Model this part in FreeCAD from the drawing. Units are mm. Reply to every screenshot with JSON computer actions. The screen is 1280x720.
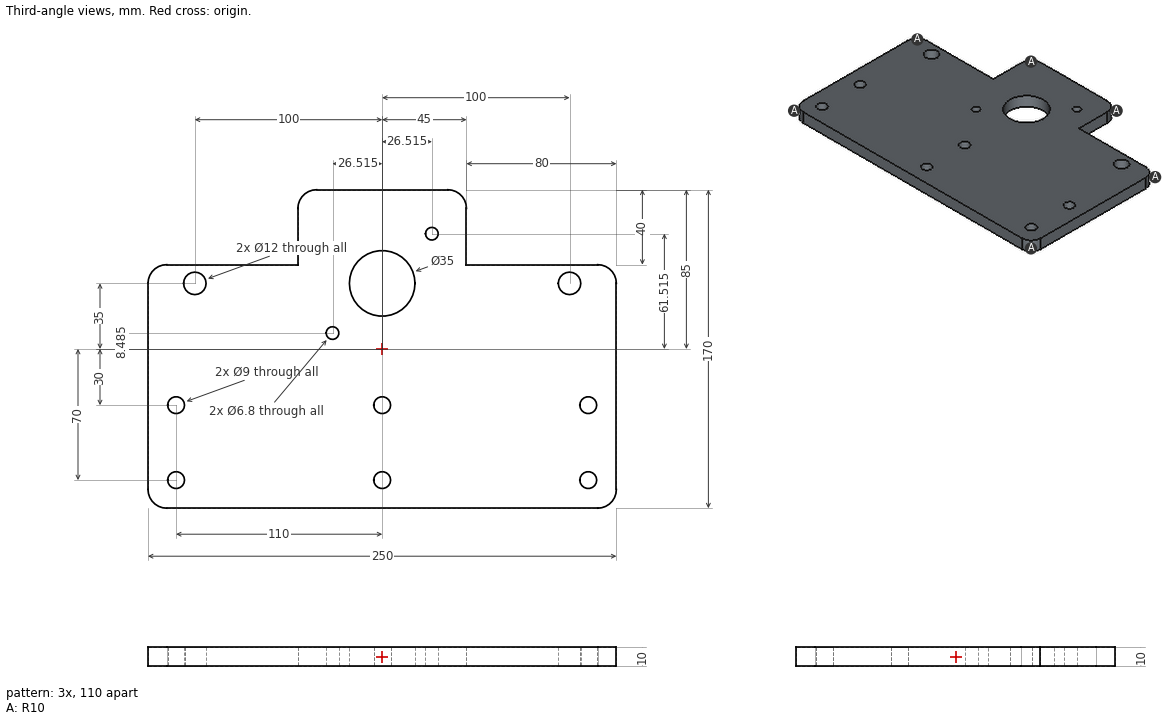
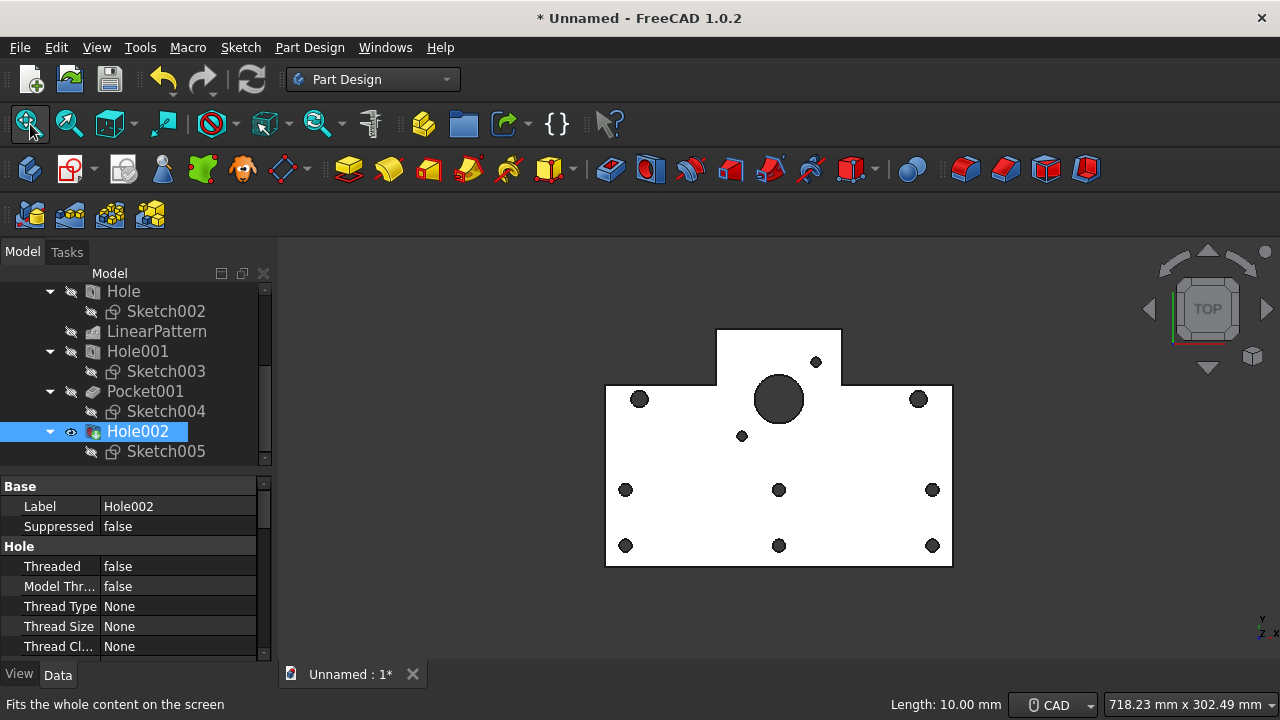
{"action": "key", "text": "1"}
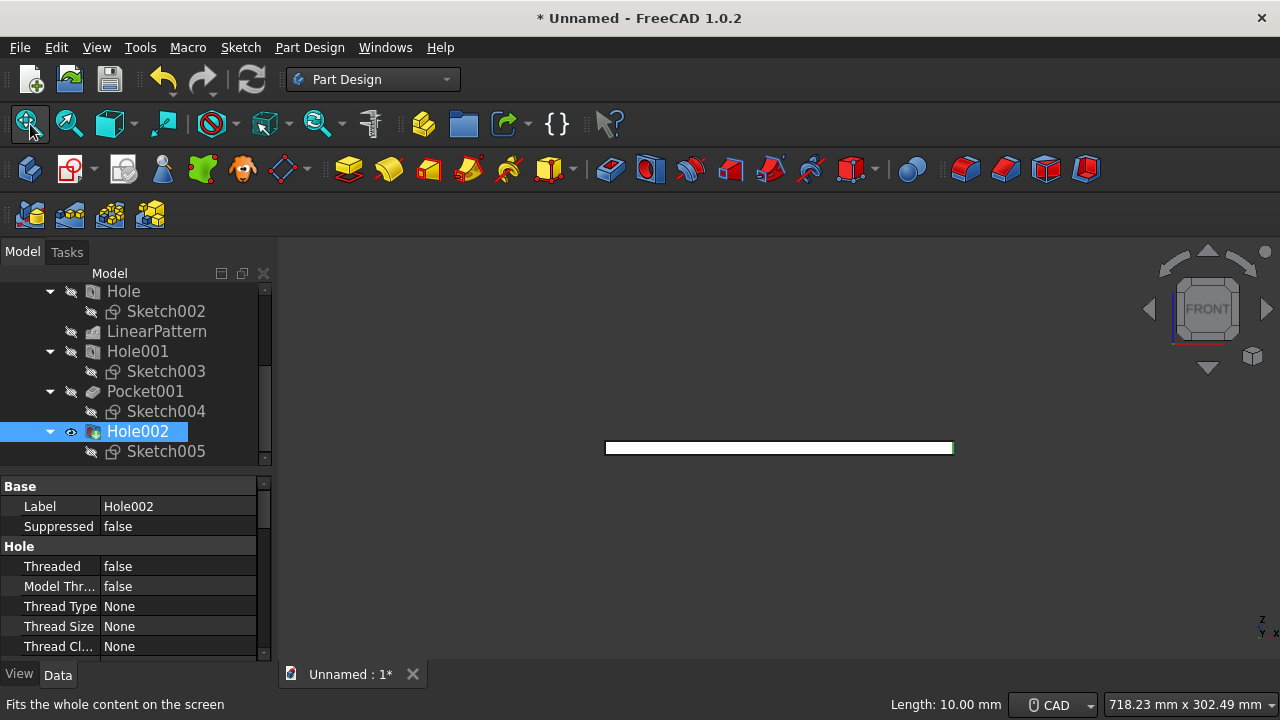
{"action": "left_click", "coordinate": [30, 124]}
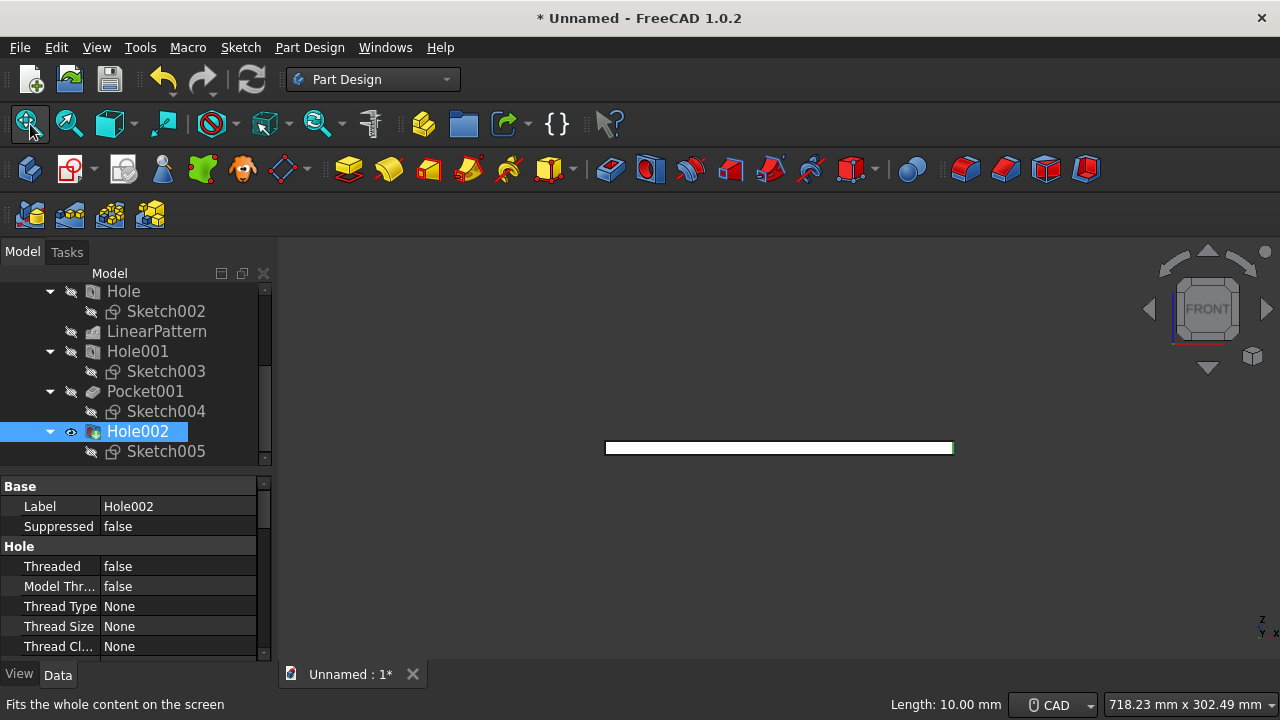
{"action": "left_click", "coordinate": [605, 447], "text": "ctrl"}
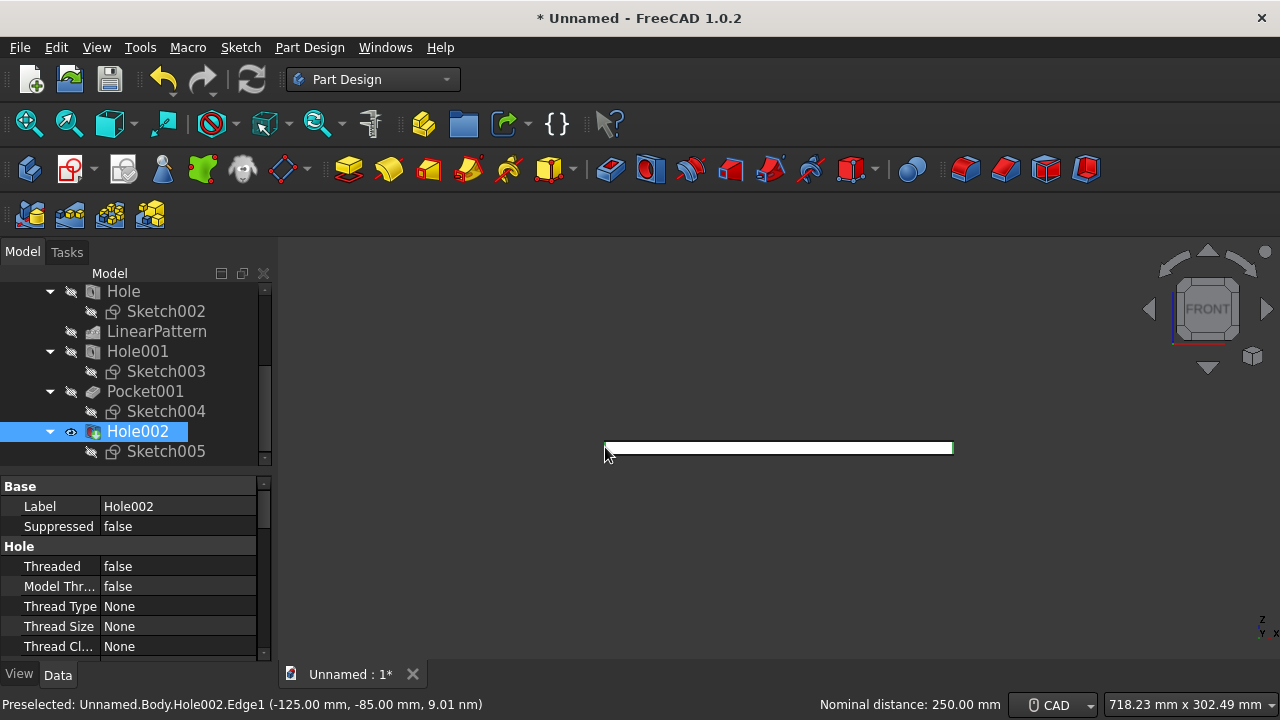
{"action": "scroll", "coordinate": [842, 447], "scroll_direction": "up", "scroll_amount": 6}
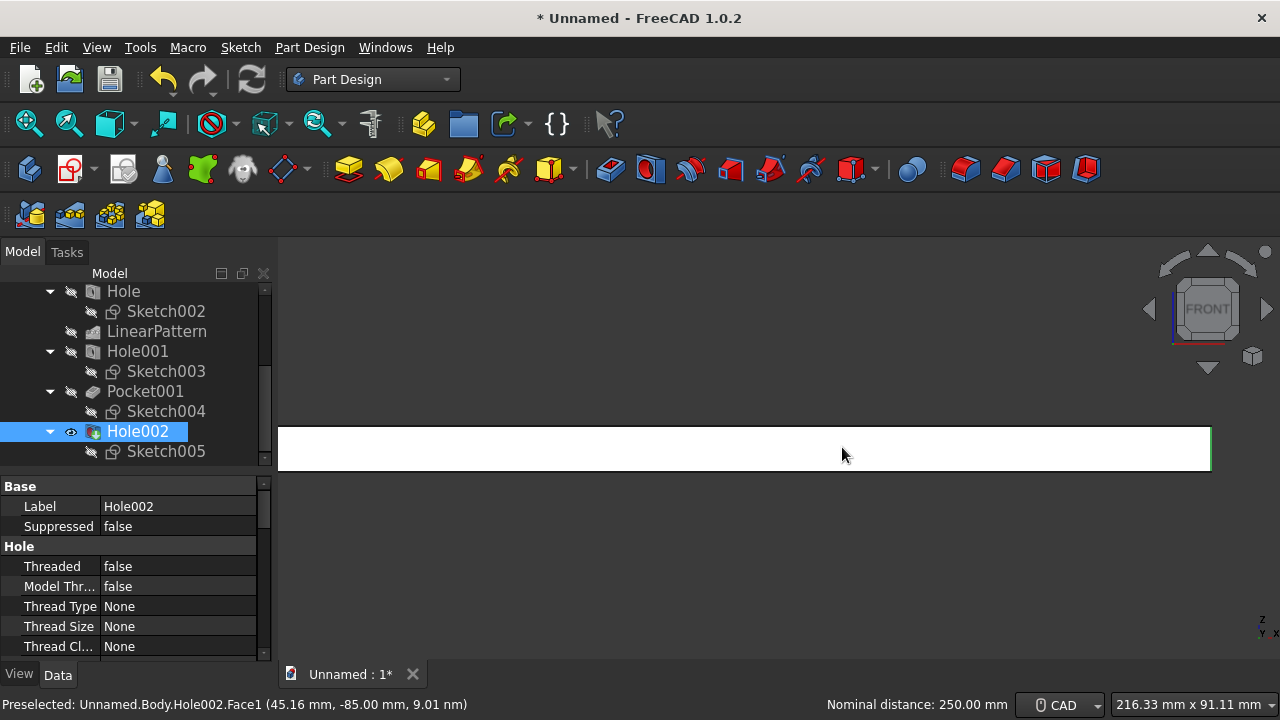
{"action": "left_click", "coordinate": [30, 124]}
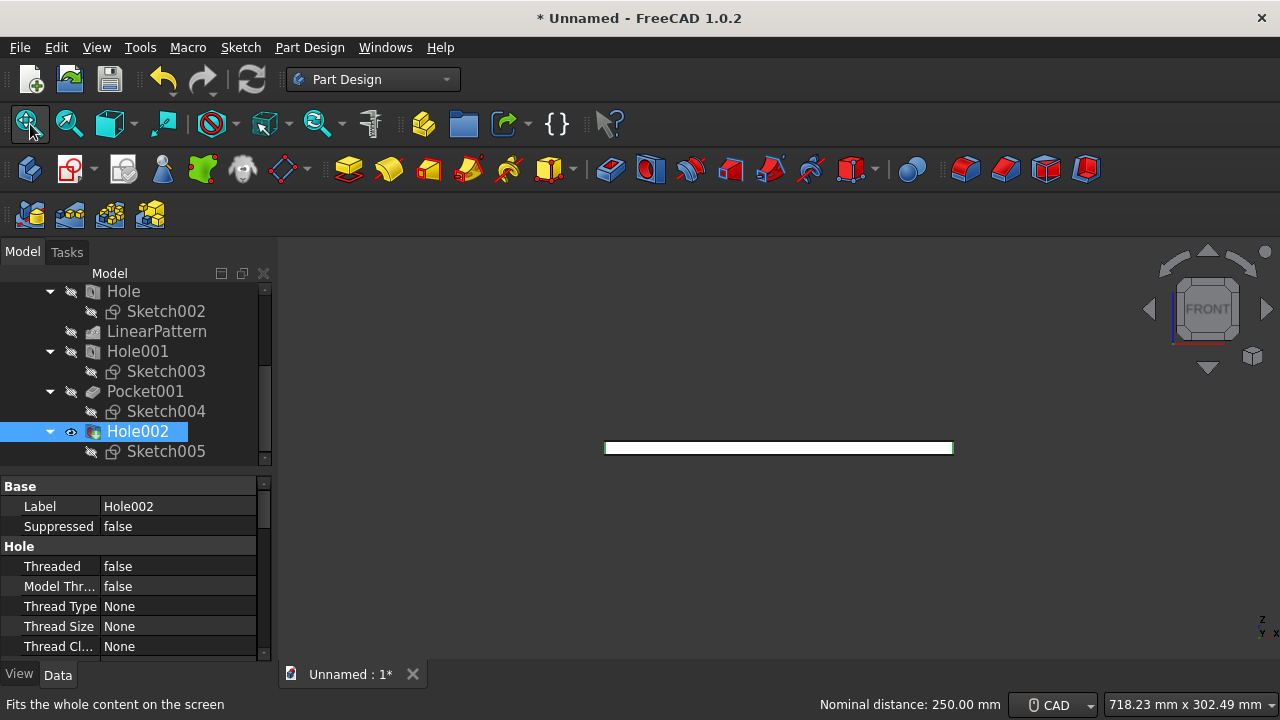
{"action": "key", "text": "3"}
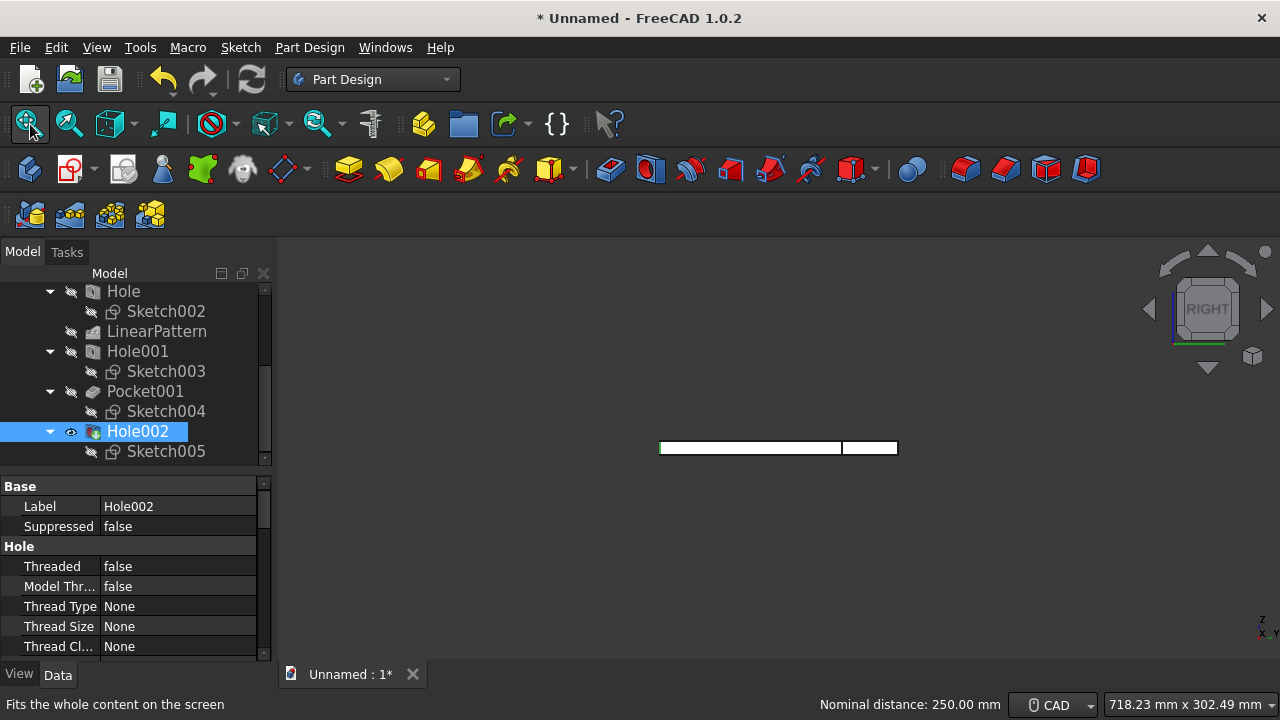
{"action": "left_click", "coordinate": [30, 124]}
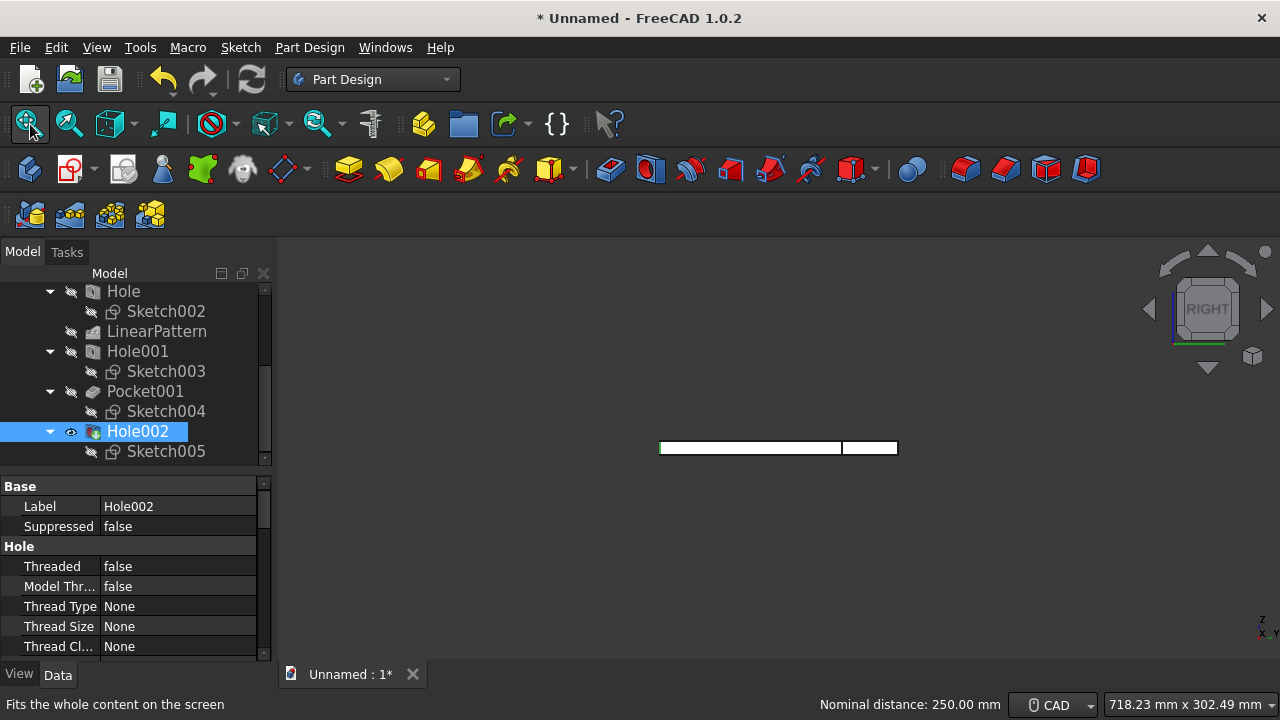
{"action": "left_click", "coordinate": [898, 447], "text": "ctrl"}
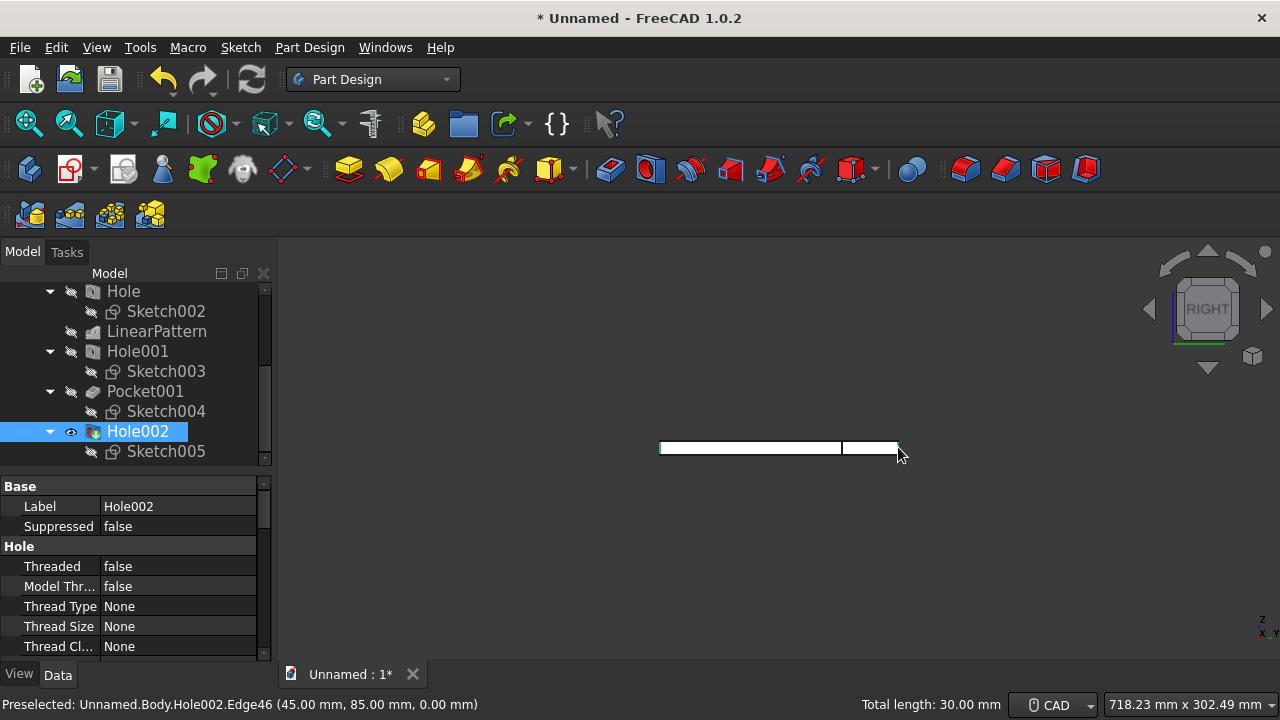
{"action": "left_click", "coordinate": [842, 447], "text": "ctrl"}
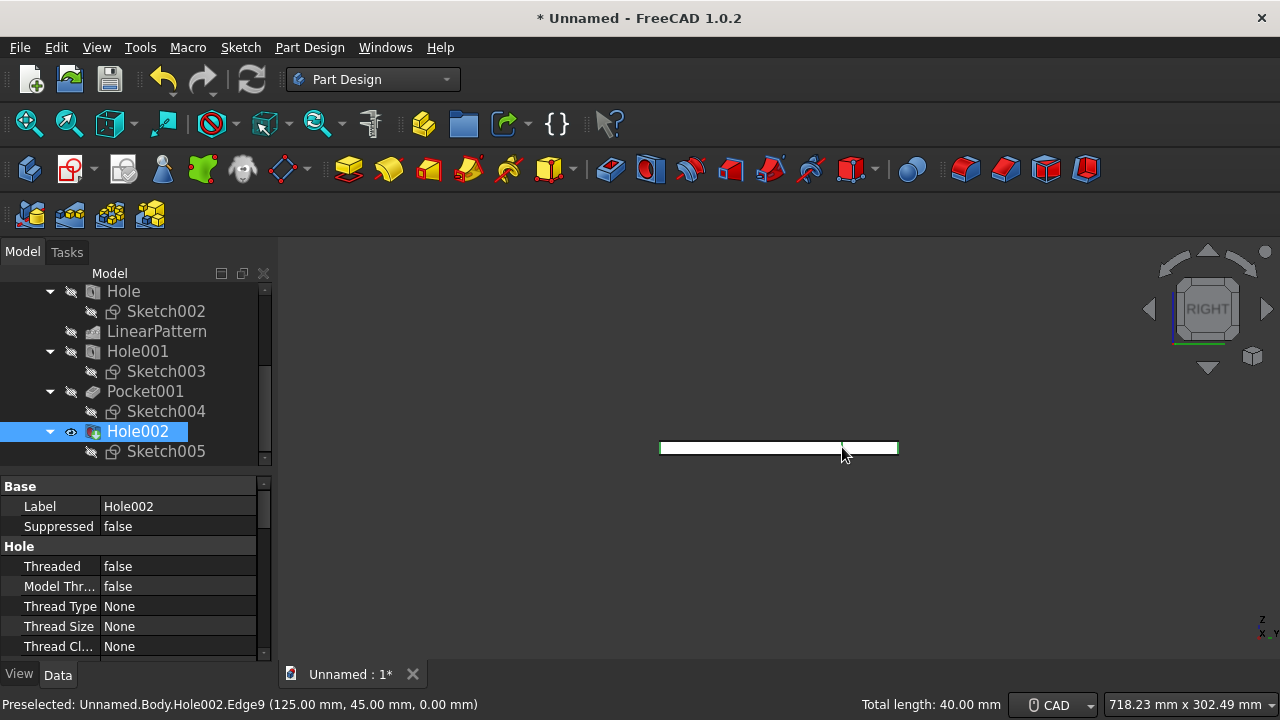
{"action": "scroll", "coordinate": [898, 447], "scroll_direction": "up", "scroll_amount": 6}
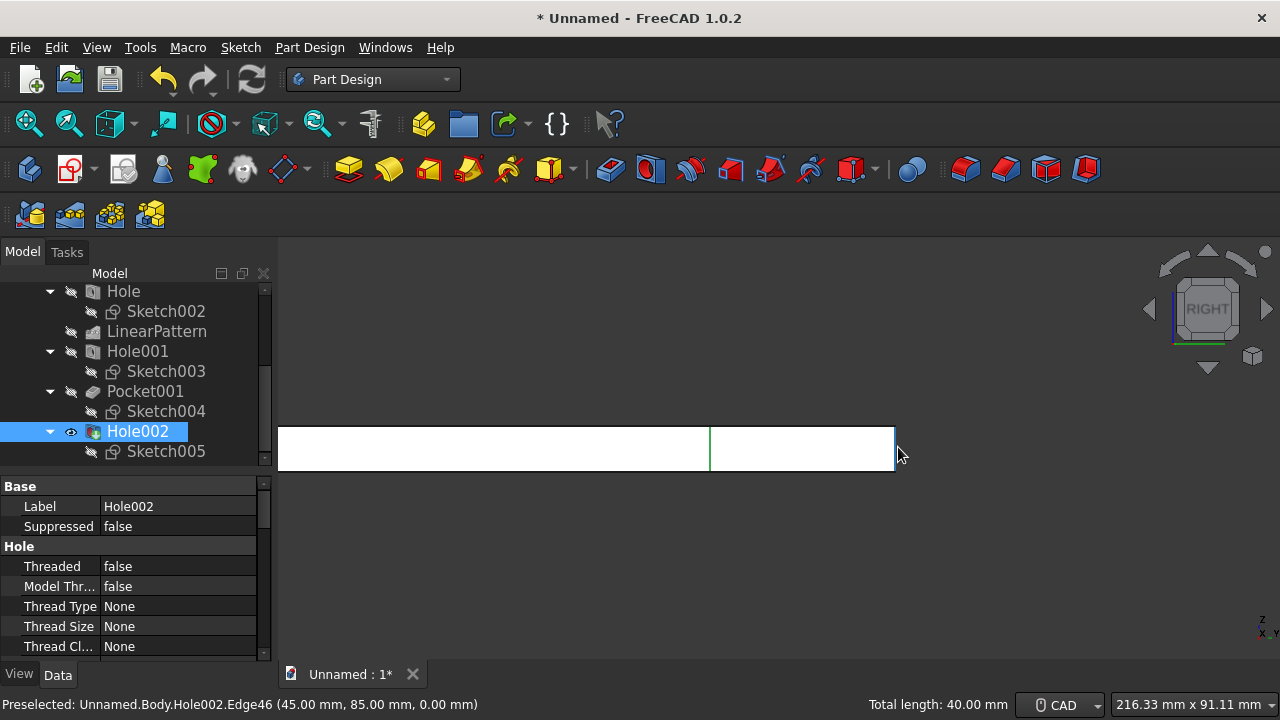
{"action": "left_click", "coordinate": [30, 124]}